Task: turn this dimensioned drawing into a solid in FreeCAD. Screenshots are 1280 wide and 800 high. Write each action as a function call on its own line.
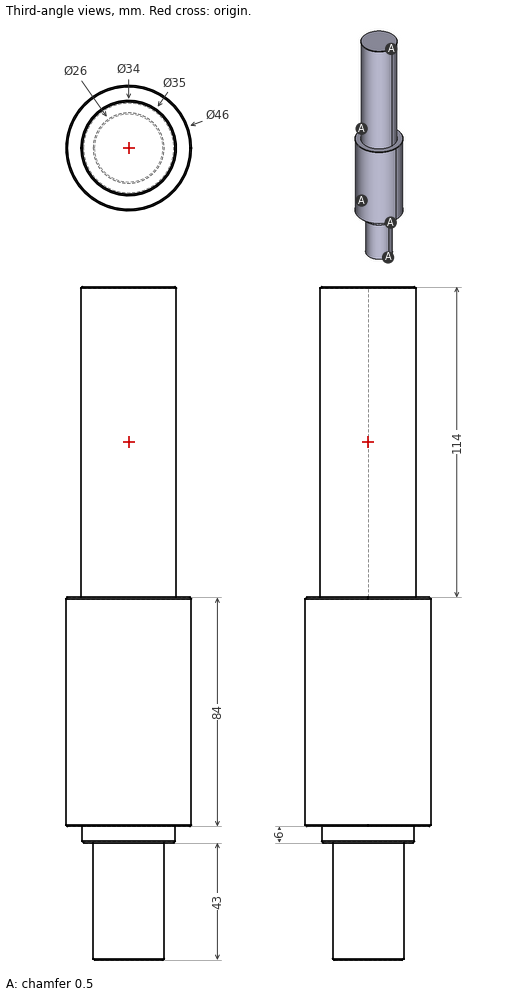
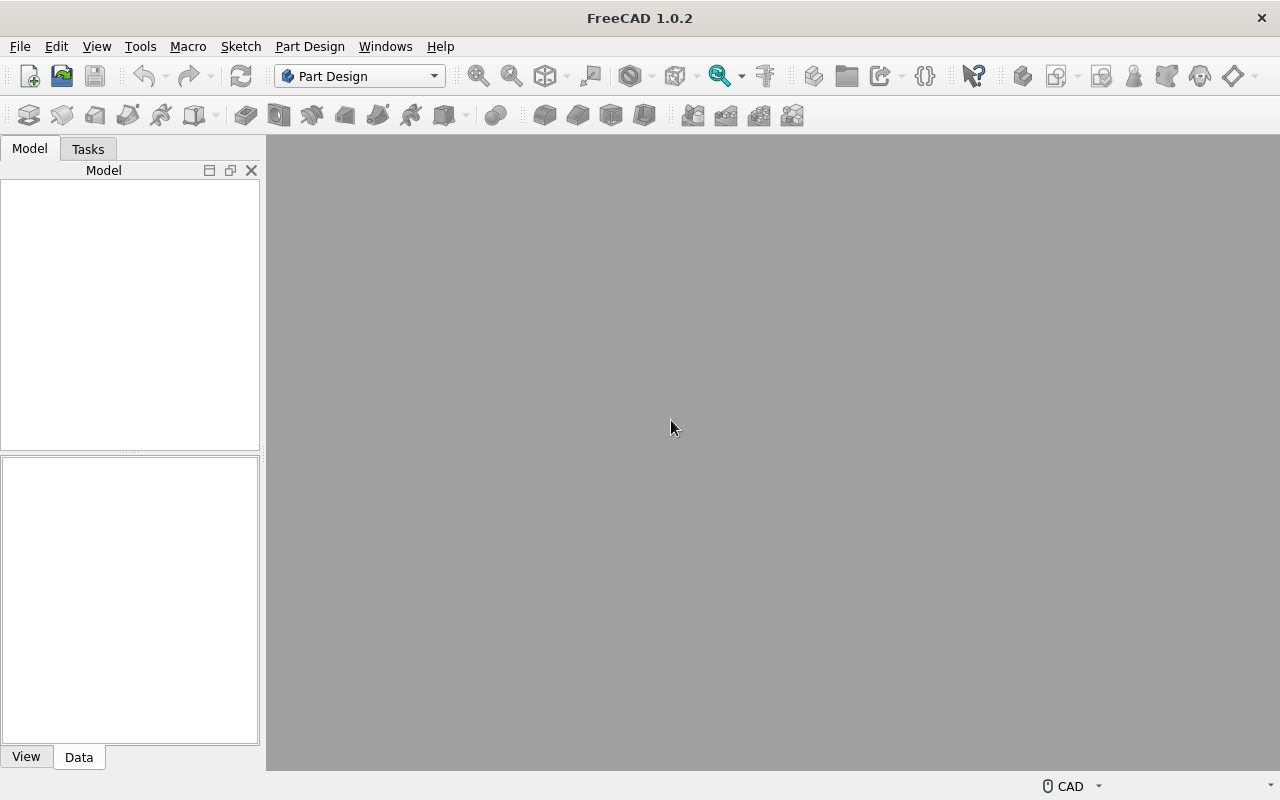
key(ctrl+n)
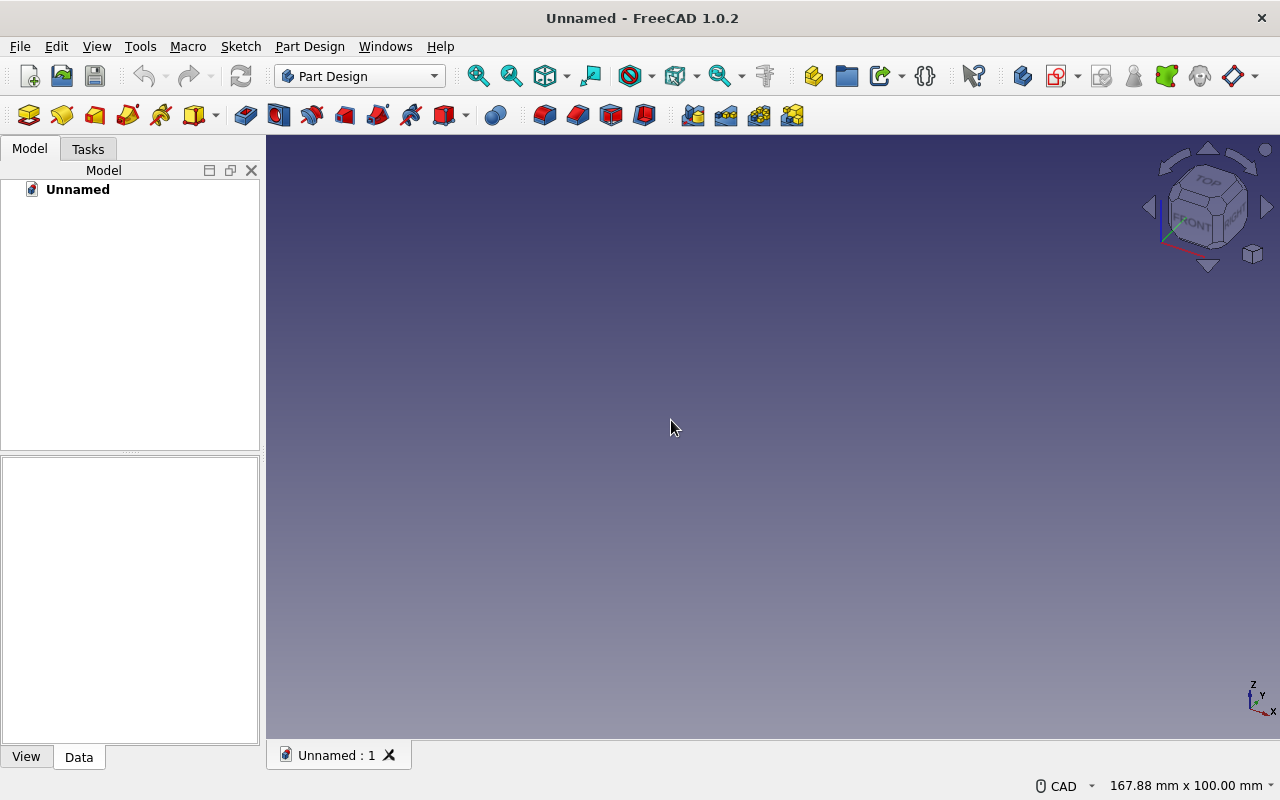
click(1056, 76)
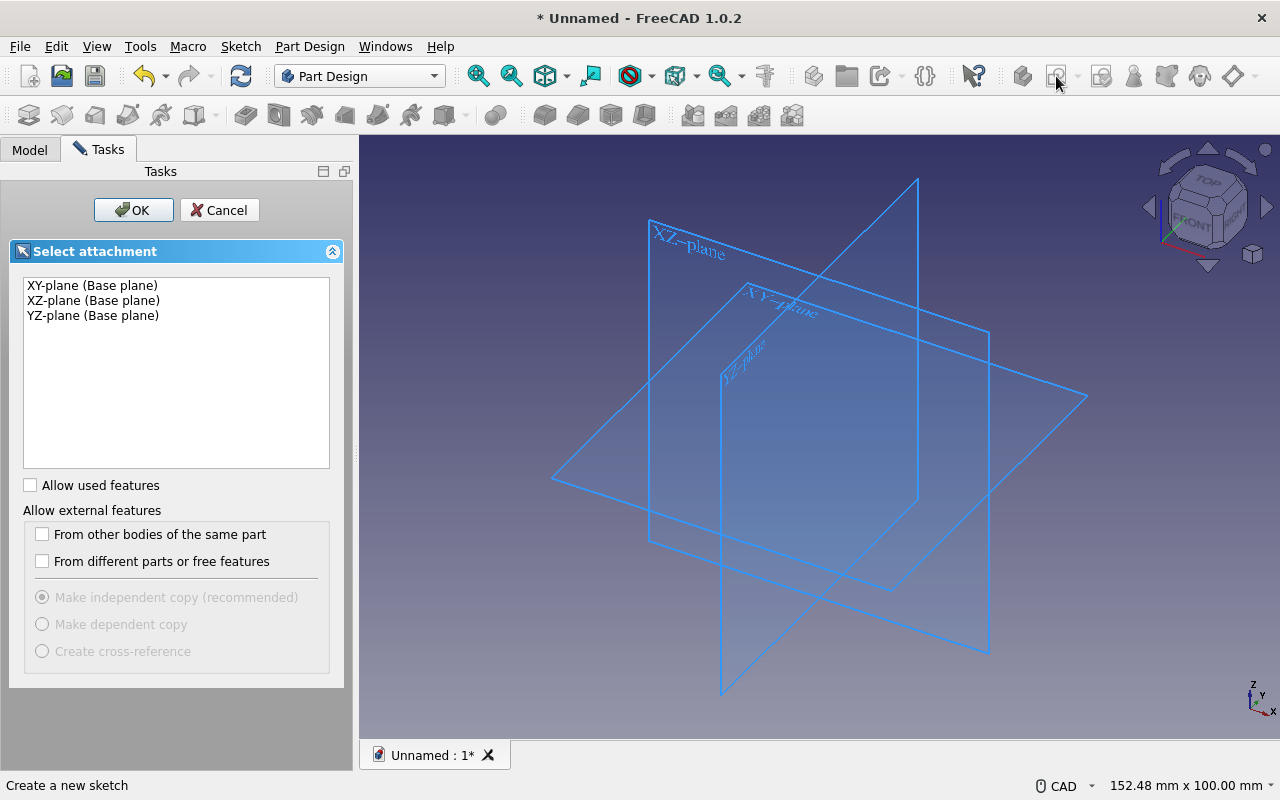
click(84, 286)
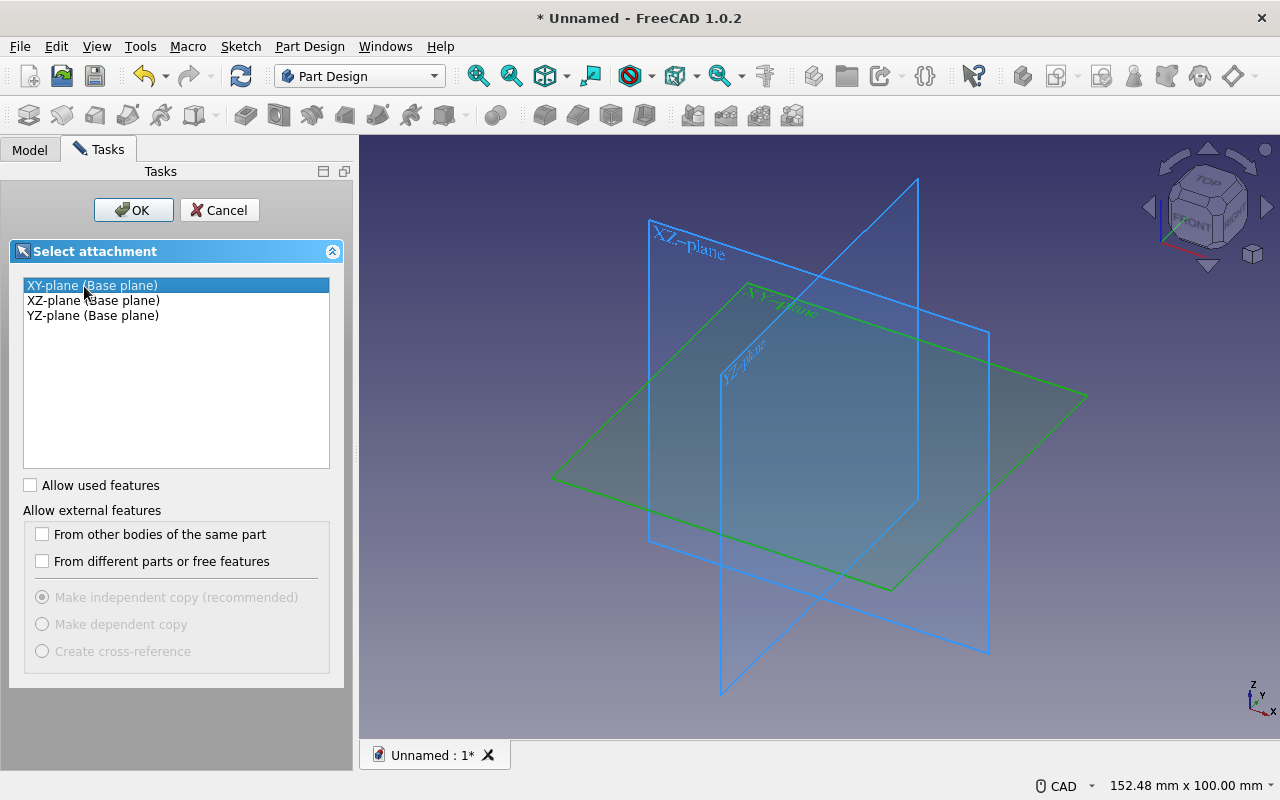
click(134, 210)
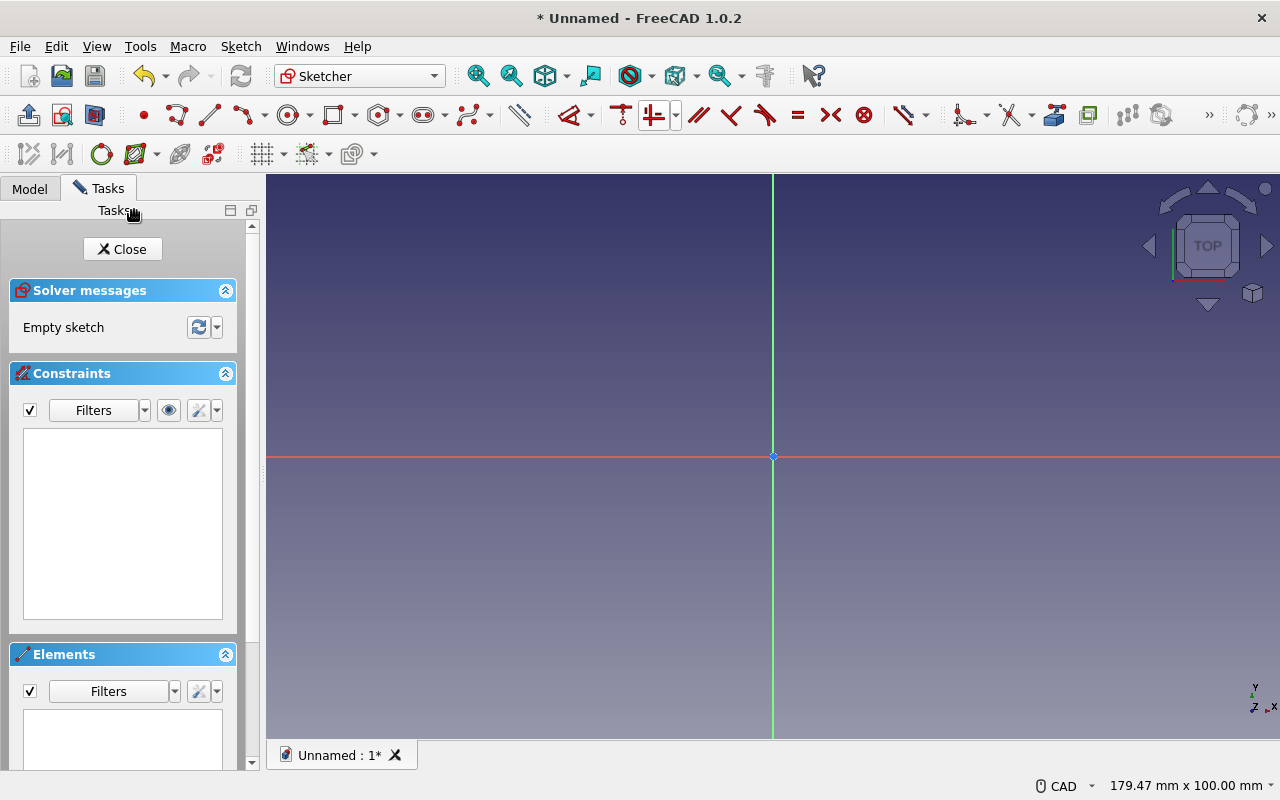
scroll(856, 456, up, 3)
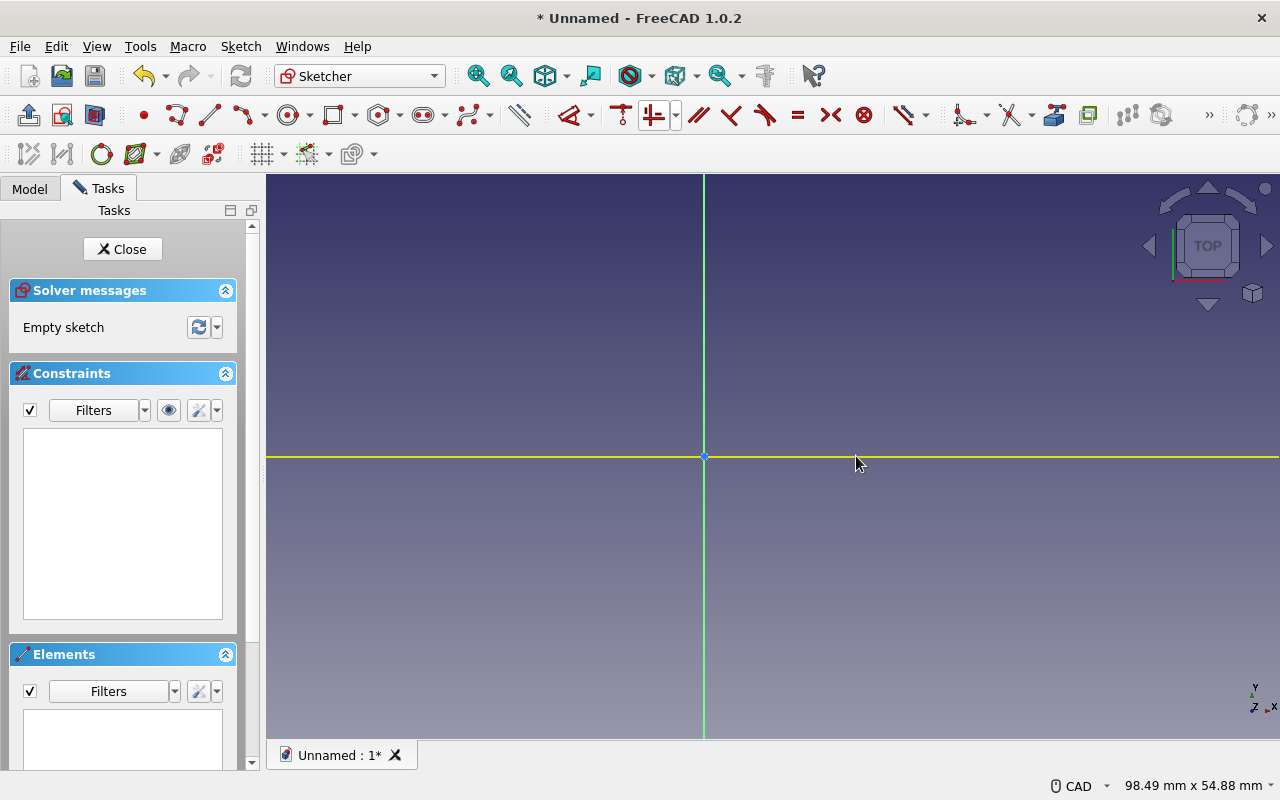
key(g)
key(c)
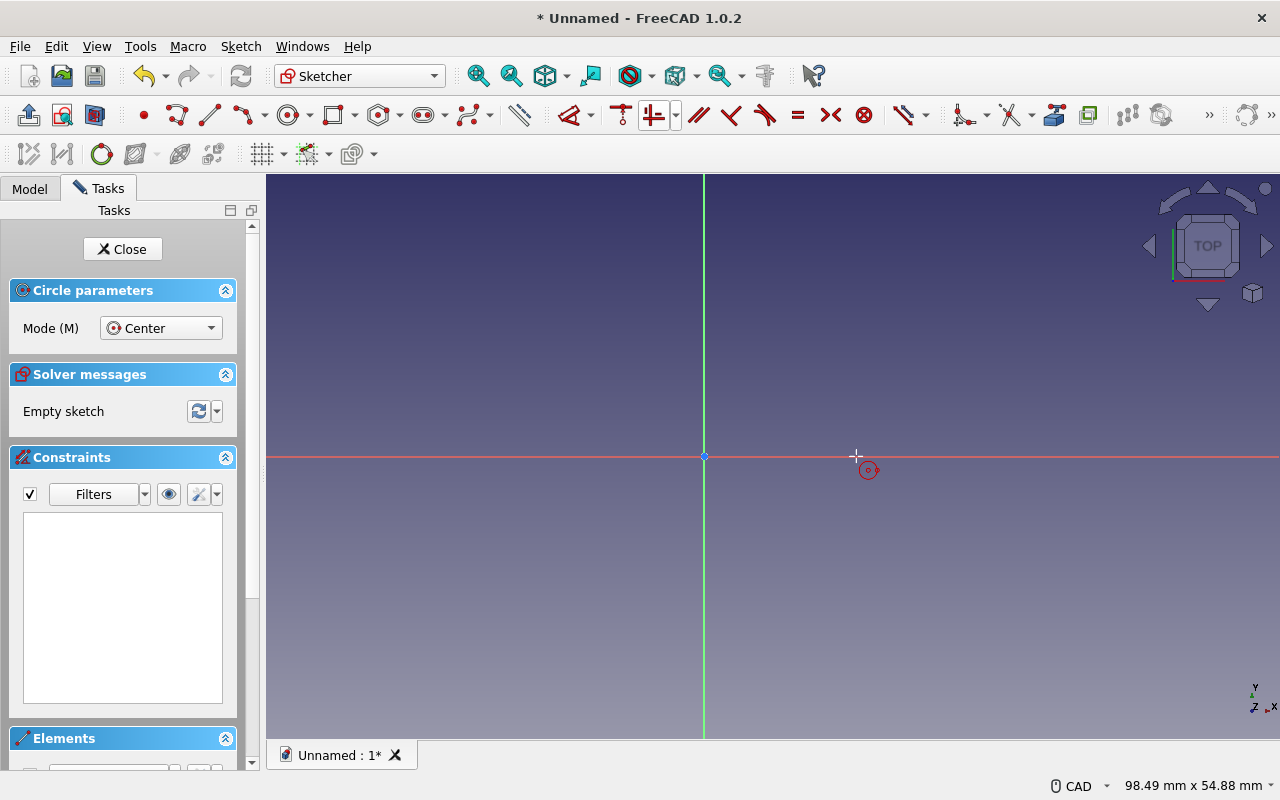
click(704, 456)
click(832, 329)
key(Escape)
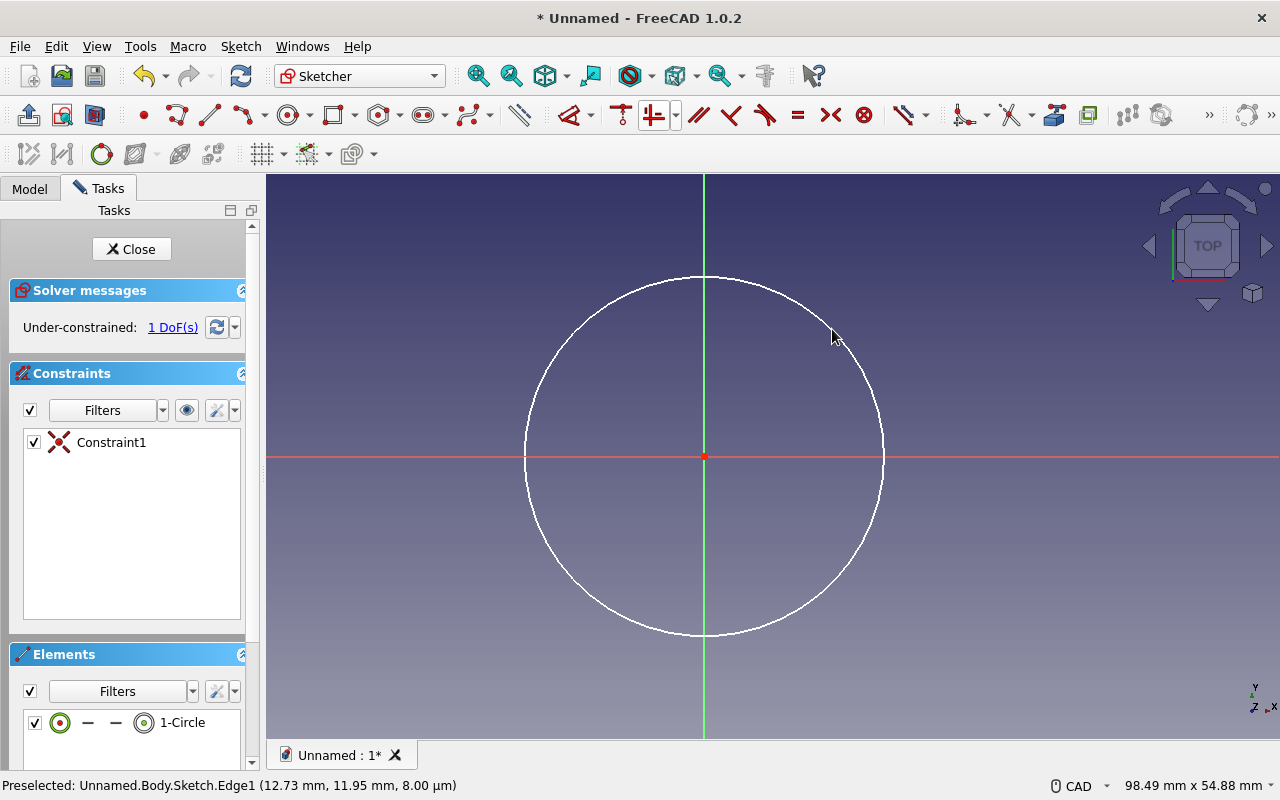
key(d)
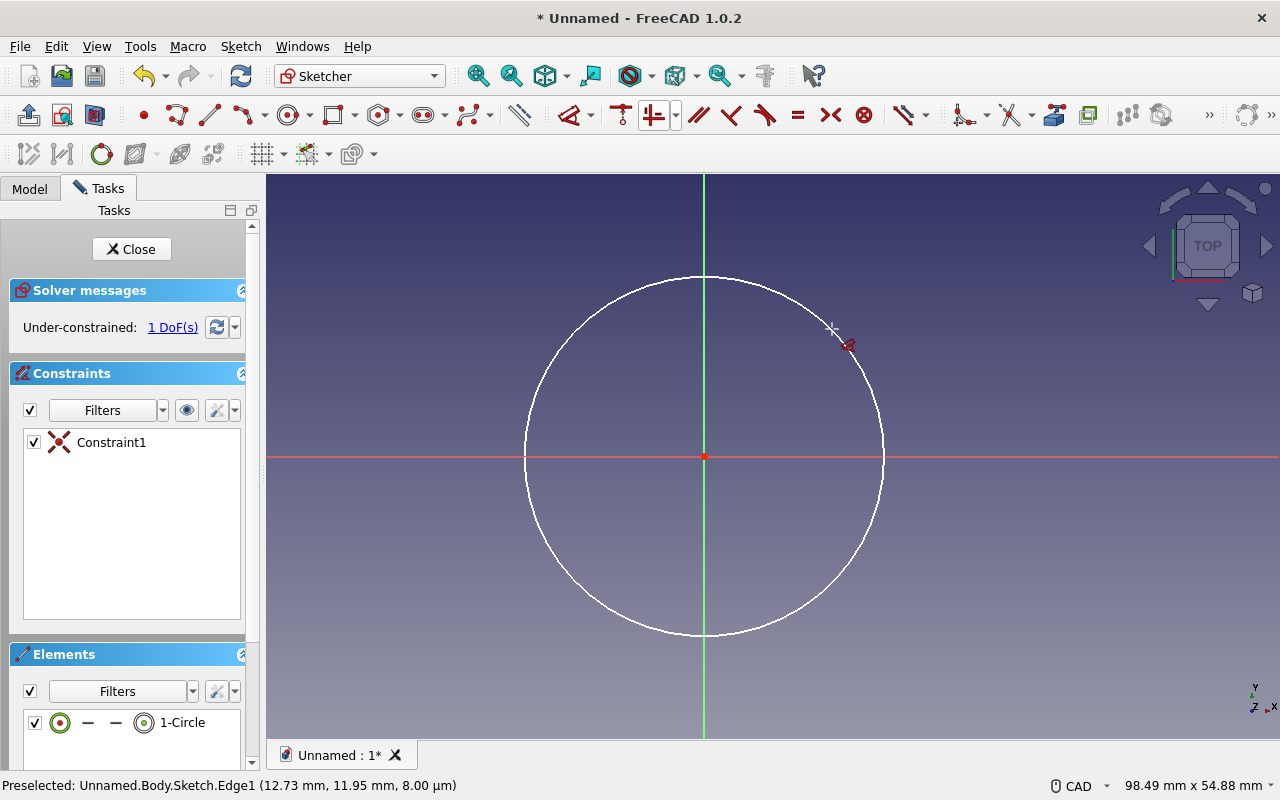
click(831, 329)
click(854, 306)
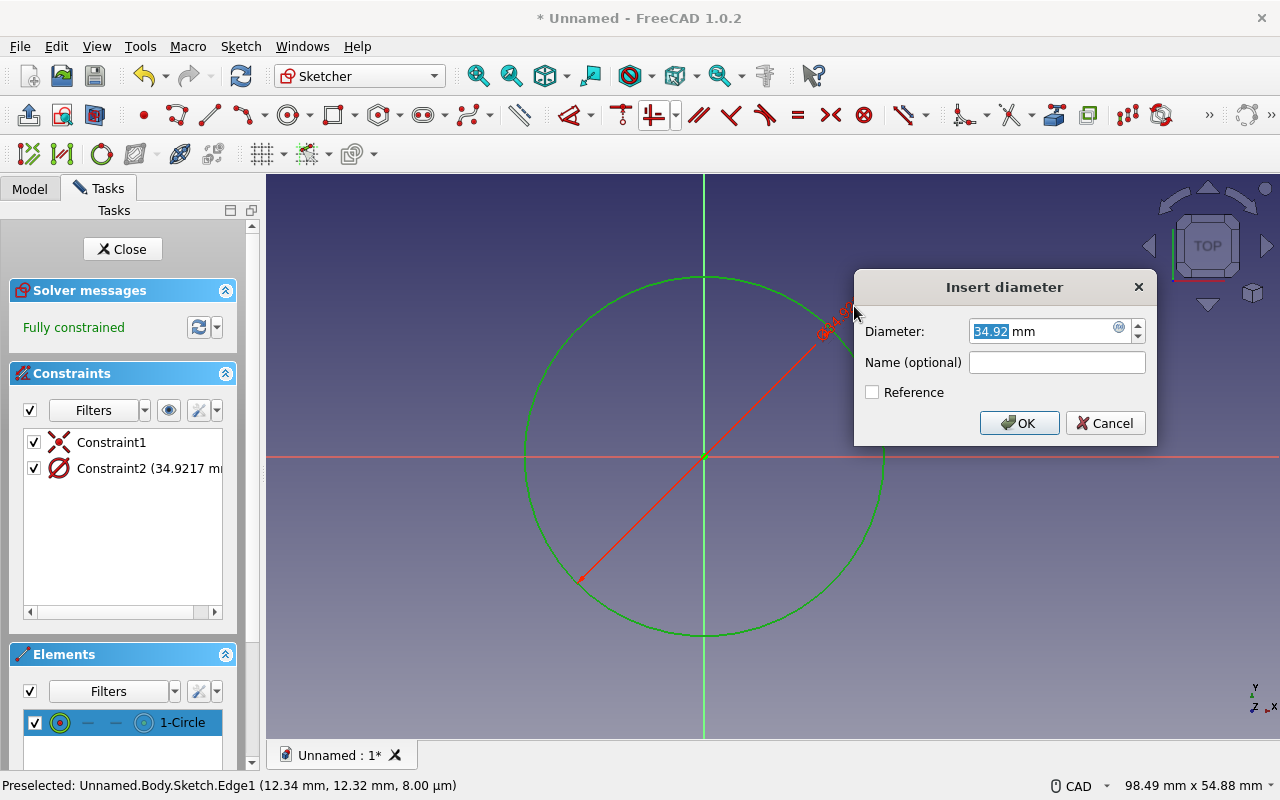
text(35)
key(Return)
key(Escape)